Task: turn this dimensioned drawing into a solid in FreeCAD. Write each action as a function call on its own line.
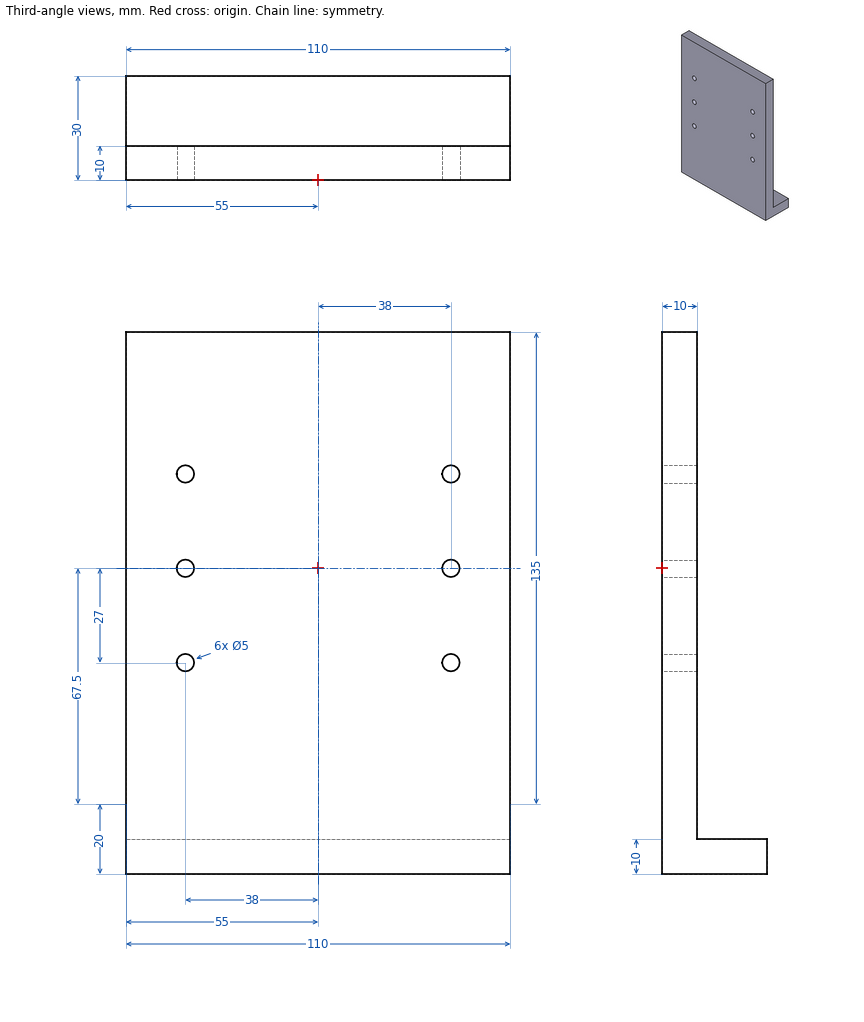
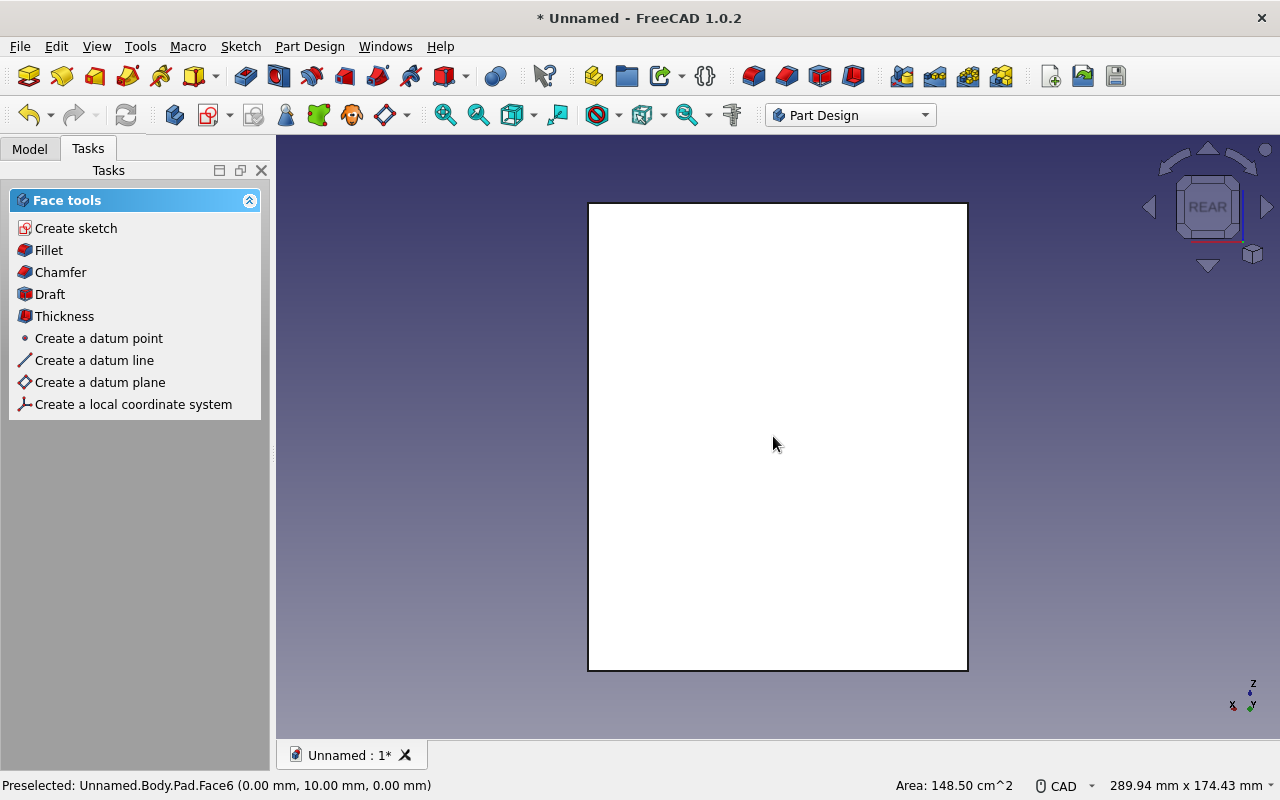
click(208, 116)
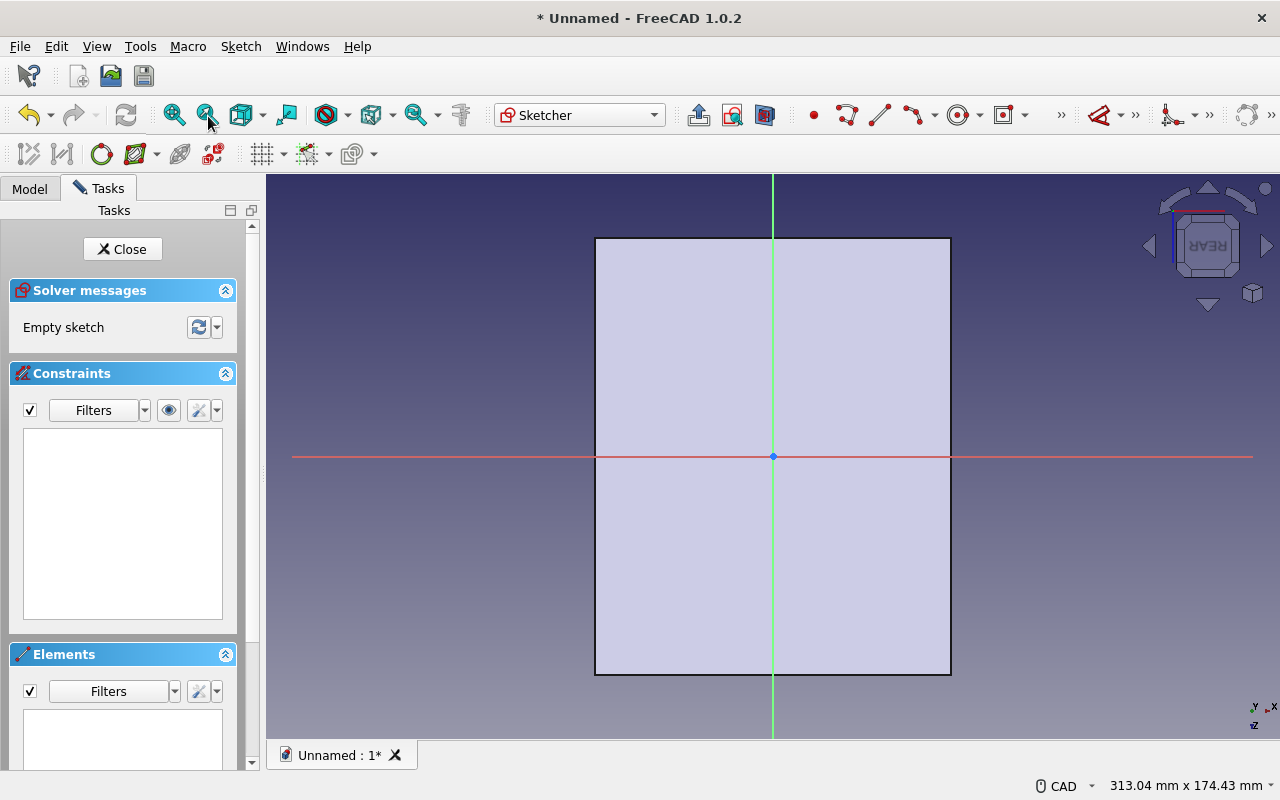
scroll(856, 457, up, 3)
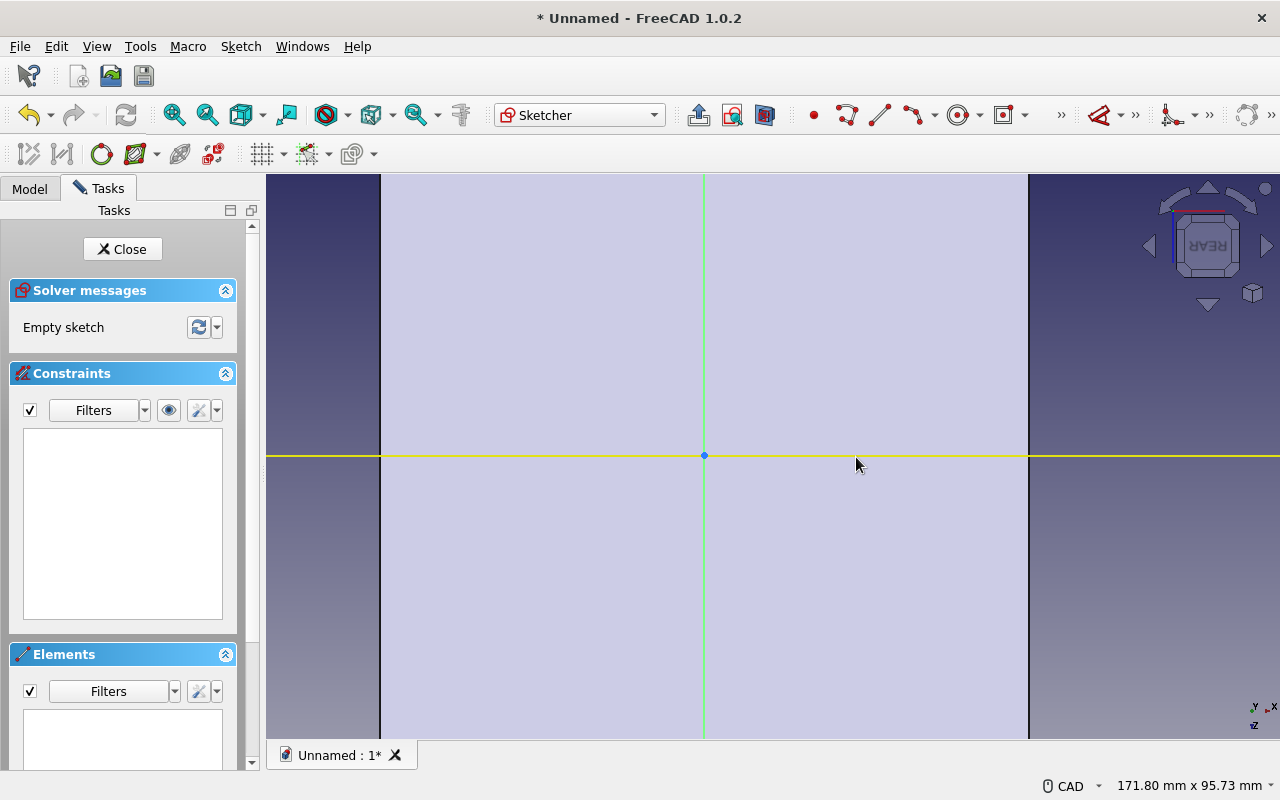
click(958, 116)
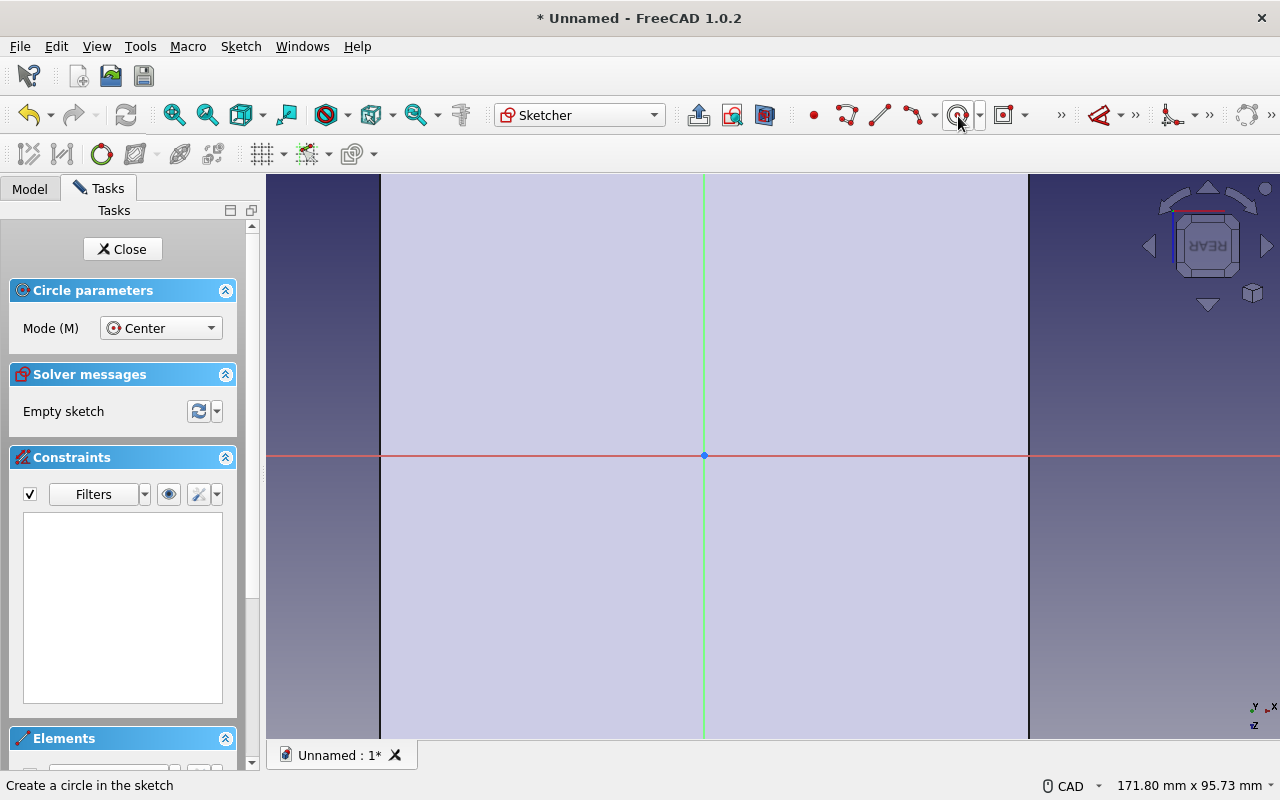
scroll(480, 296, up, 3)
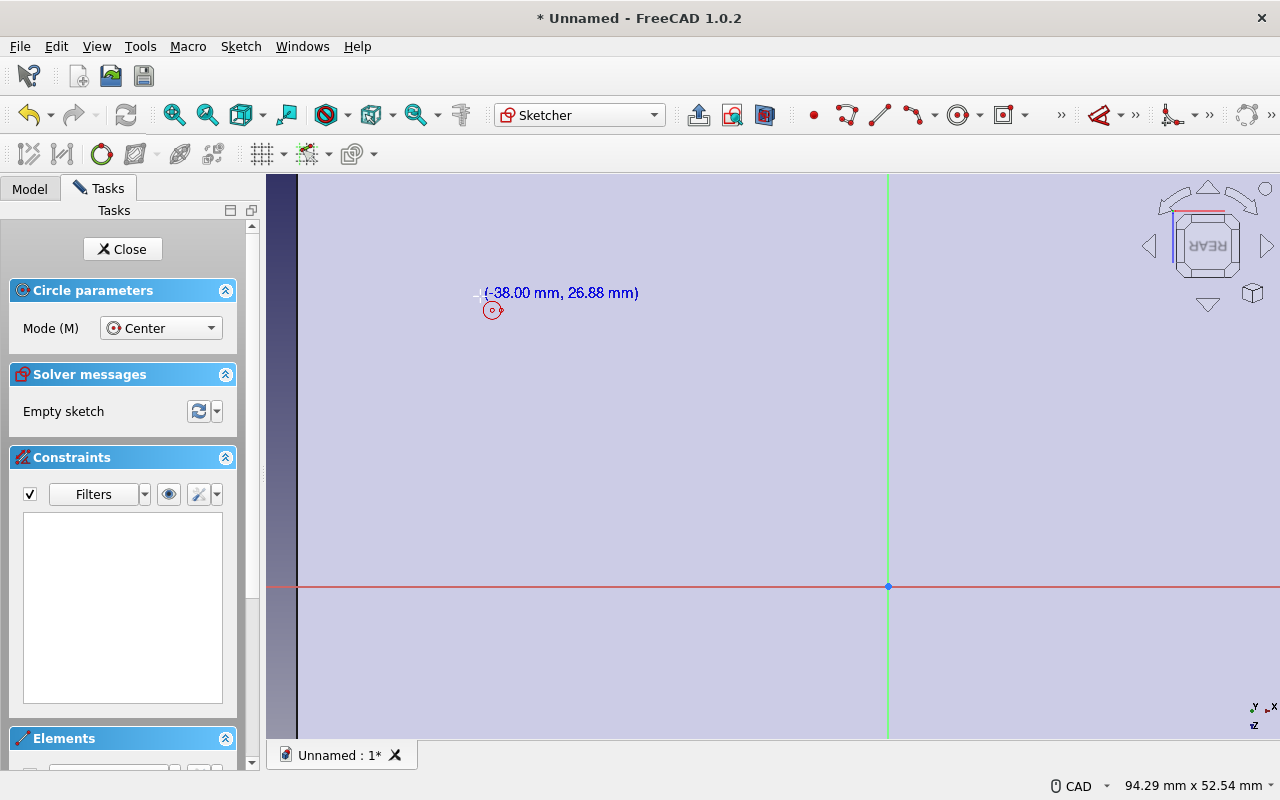
click(480, 296)
click(499, 277)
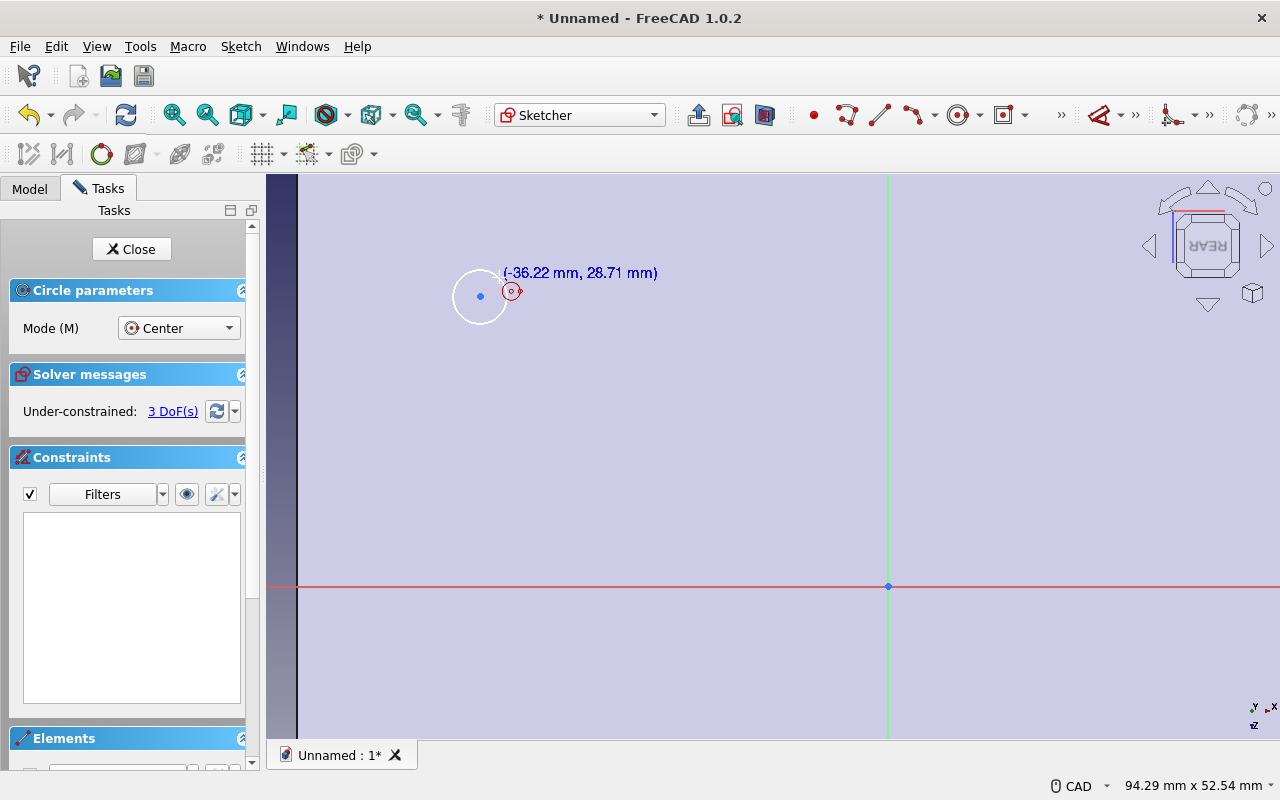
click(480, 587)
click(499, 568)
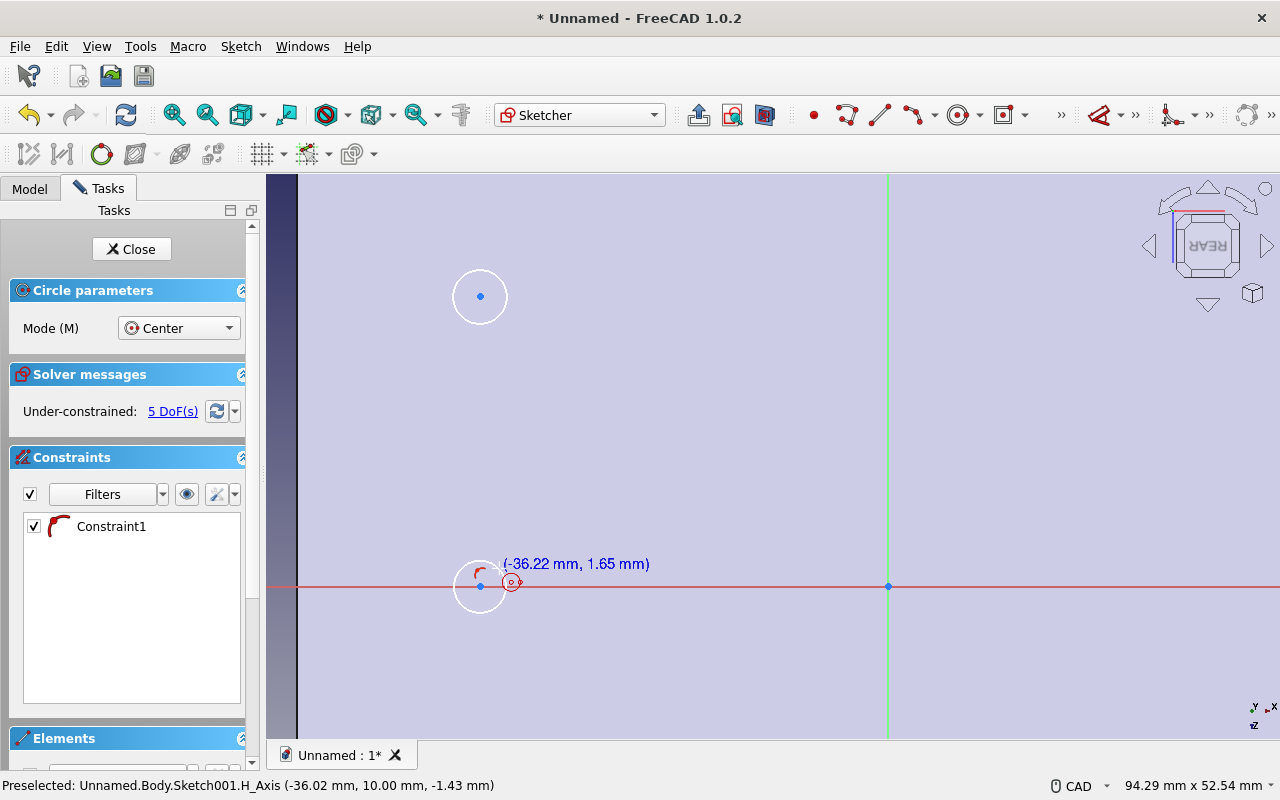
scroll(481, 298, down, 3)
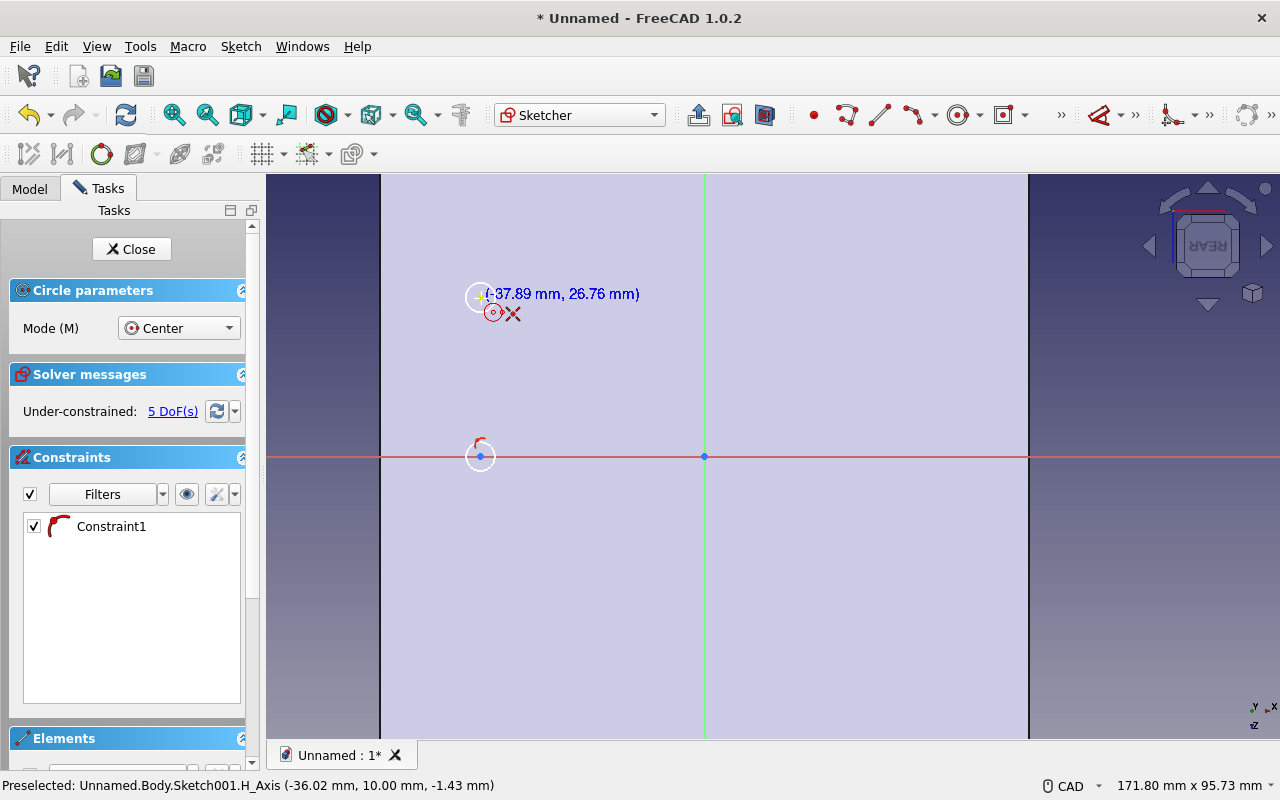
scroll(929, 457, up, 3)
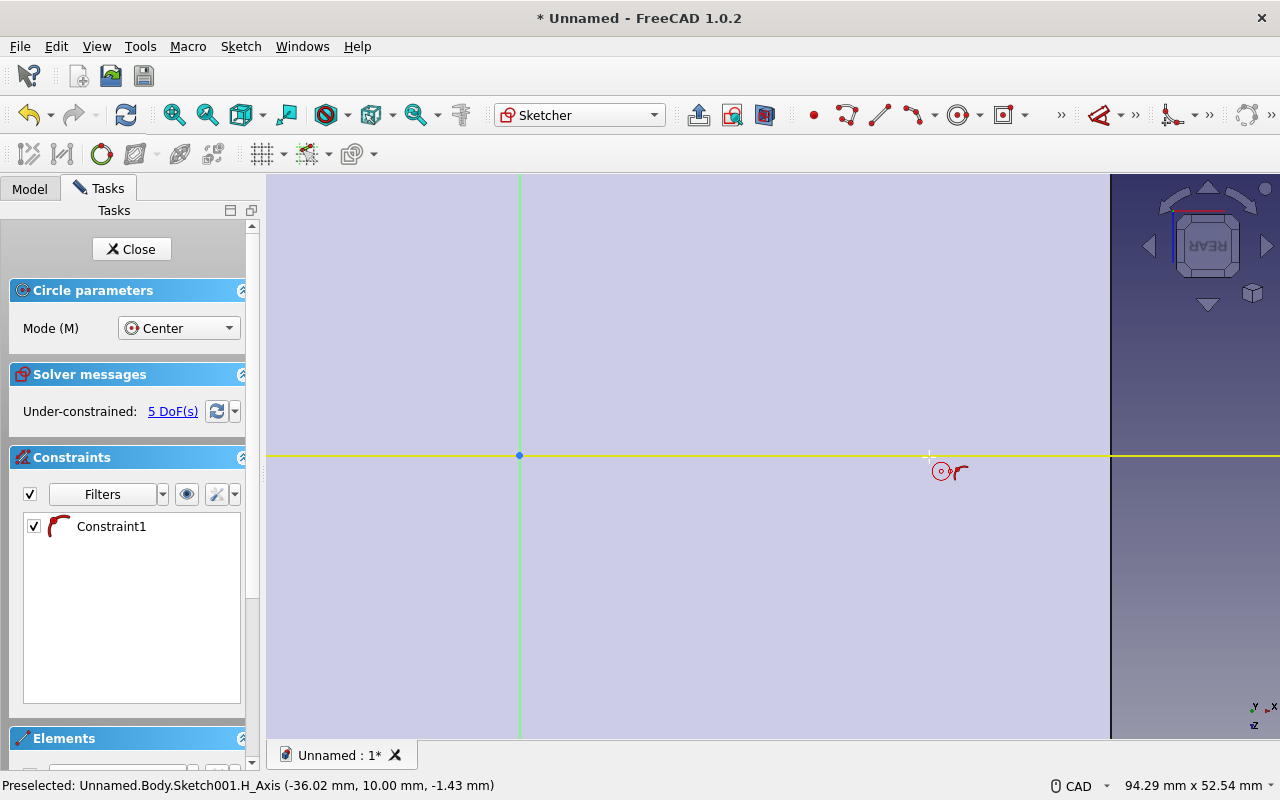
click(928, 456)
click(948, 437)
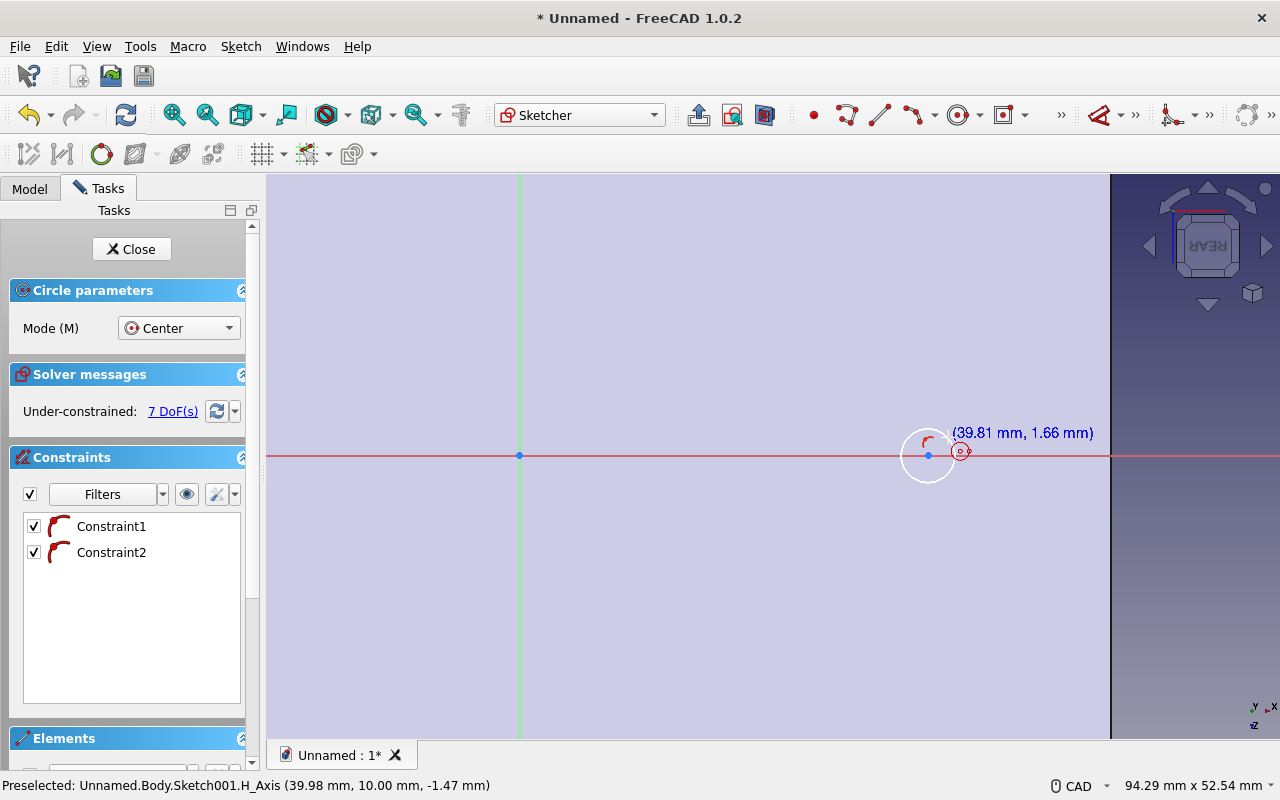
scroll(929, 457, down, 3)